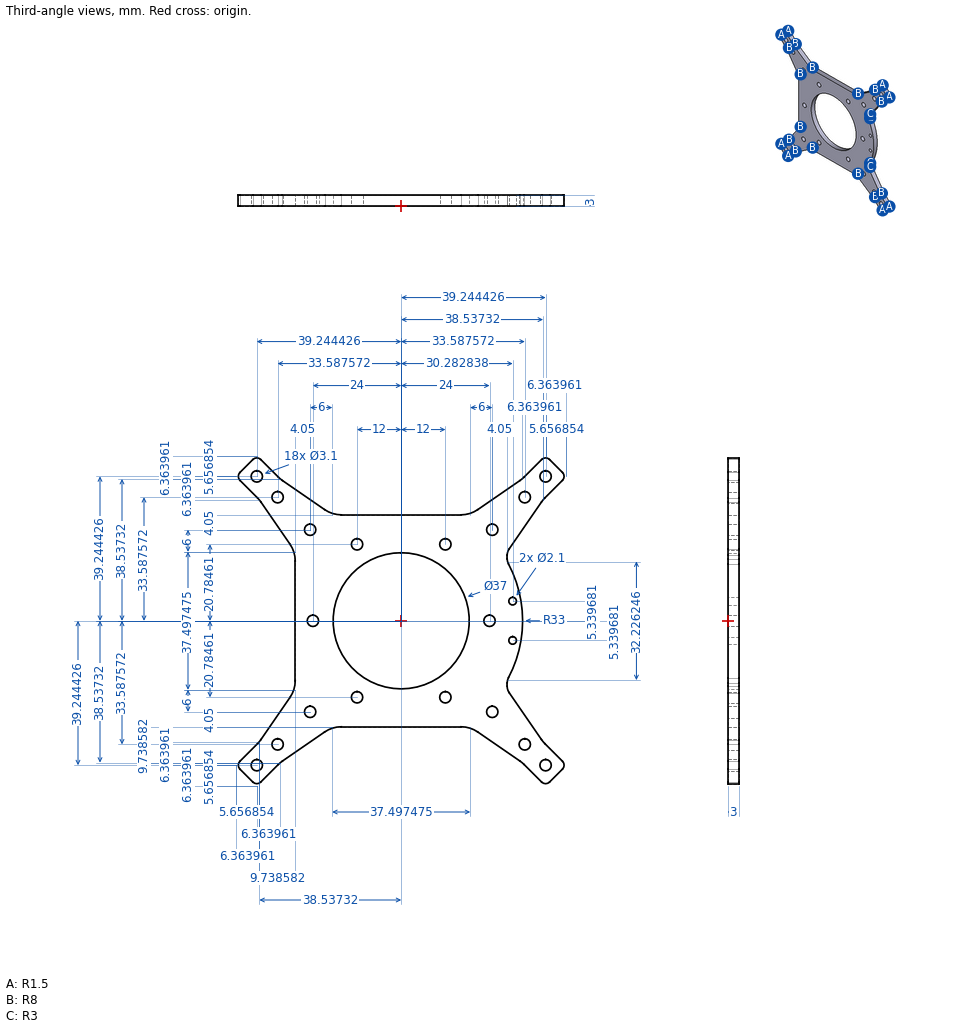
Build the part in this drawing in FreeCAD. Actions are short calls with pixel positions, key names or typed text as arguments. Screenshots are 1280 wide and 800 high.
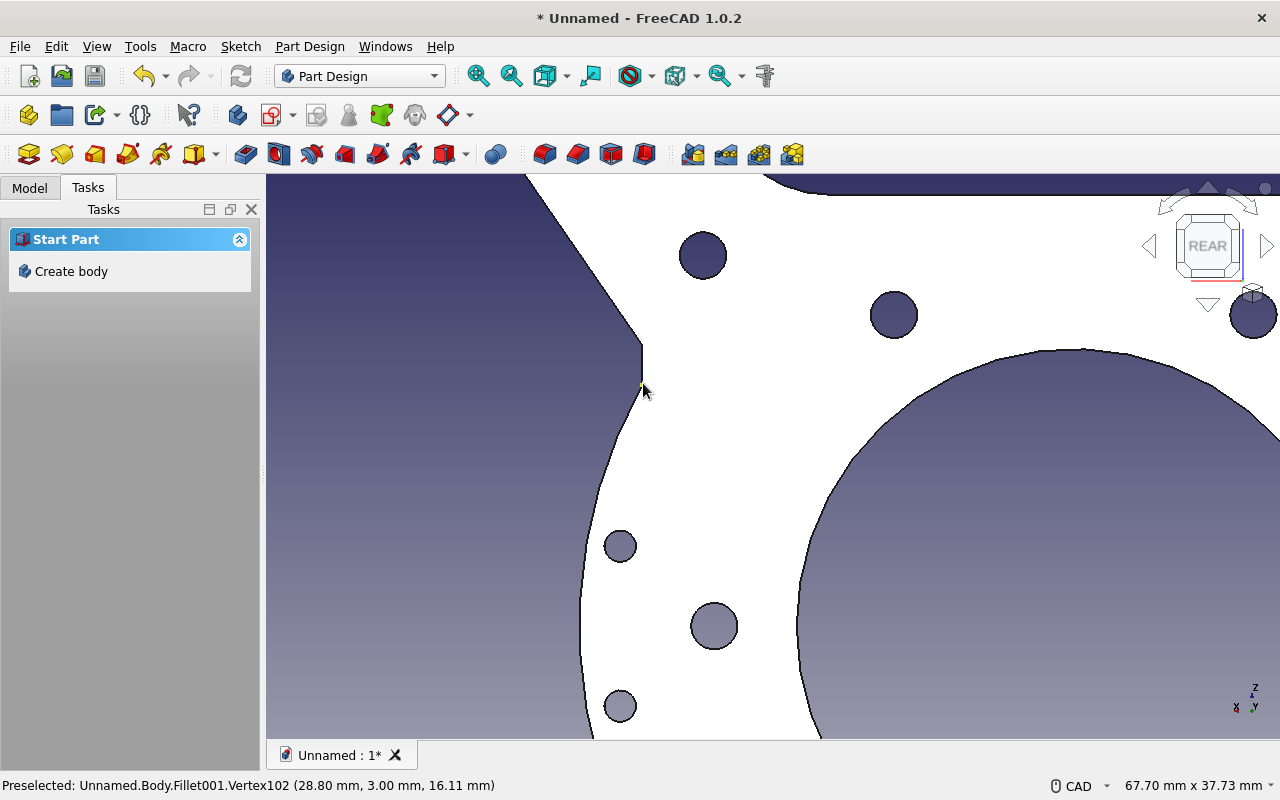
key(v)
key(f)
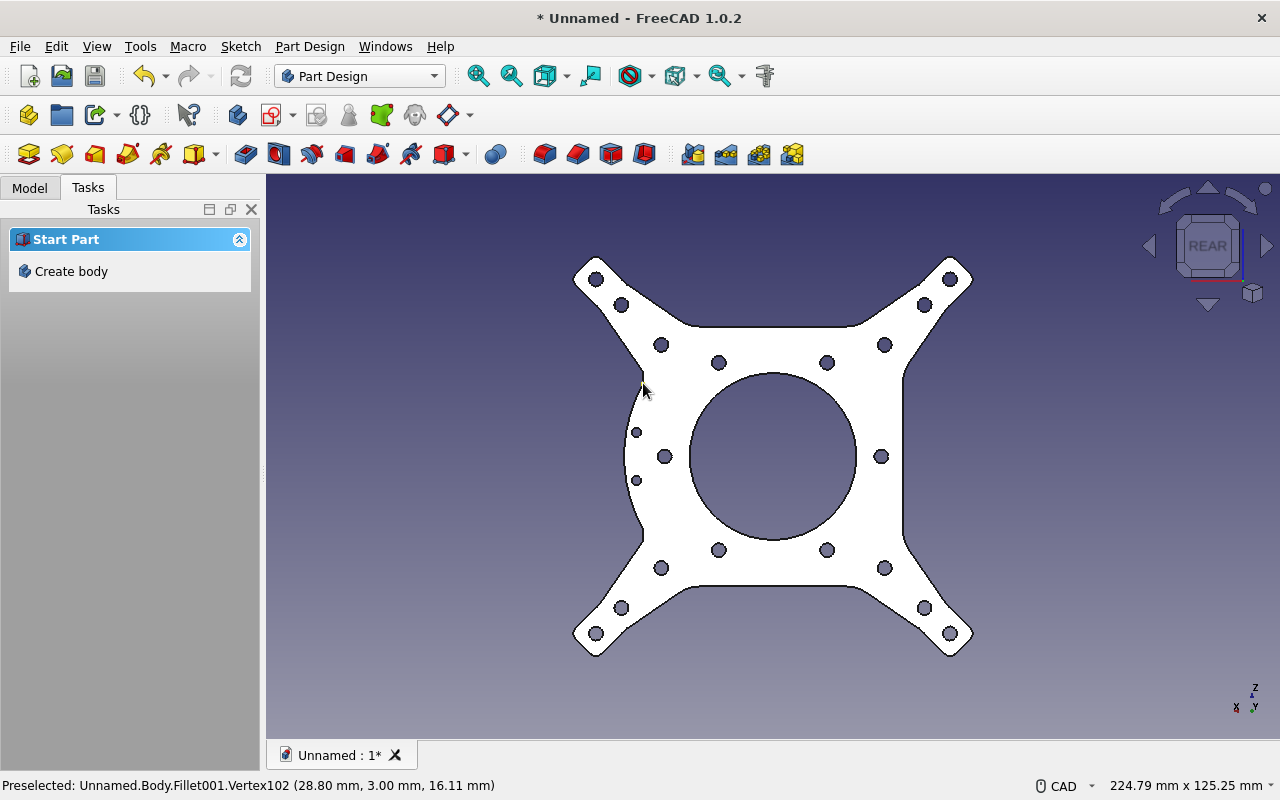
key(6)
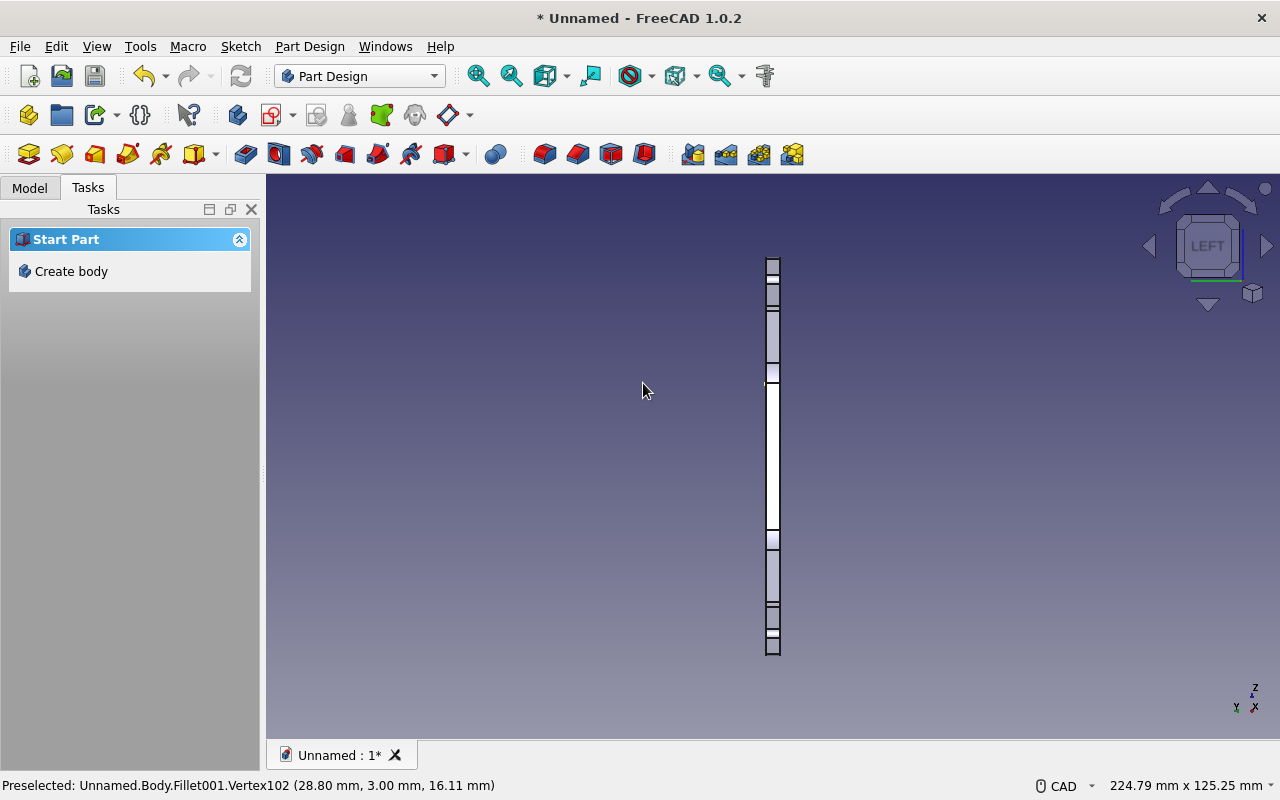
scroll(773, 383, up, 6)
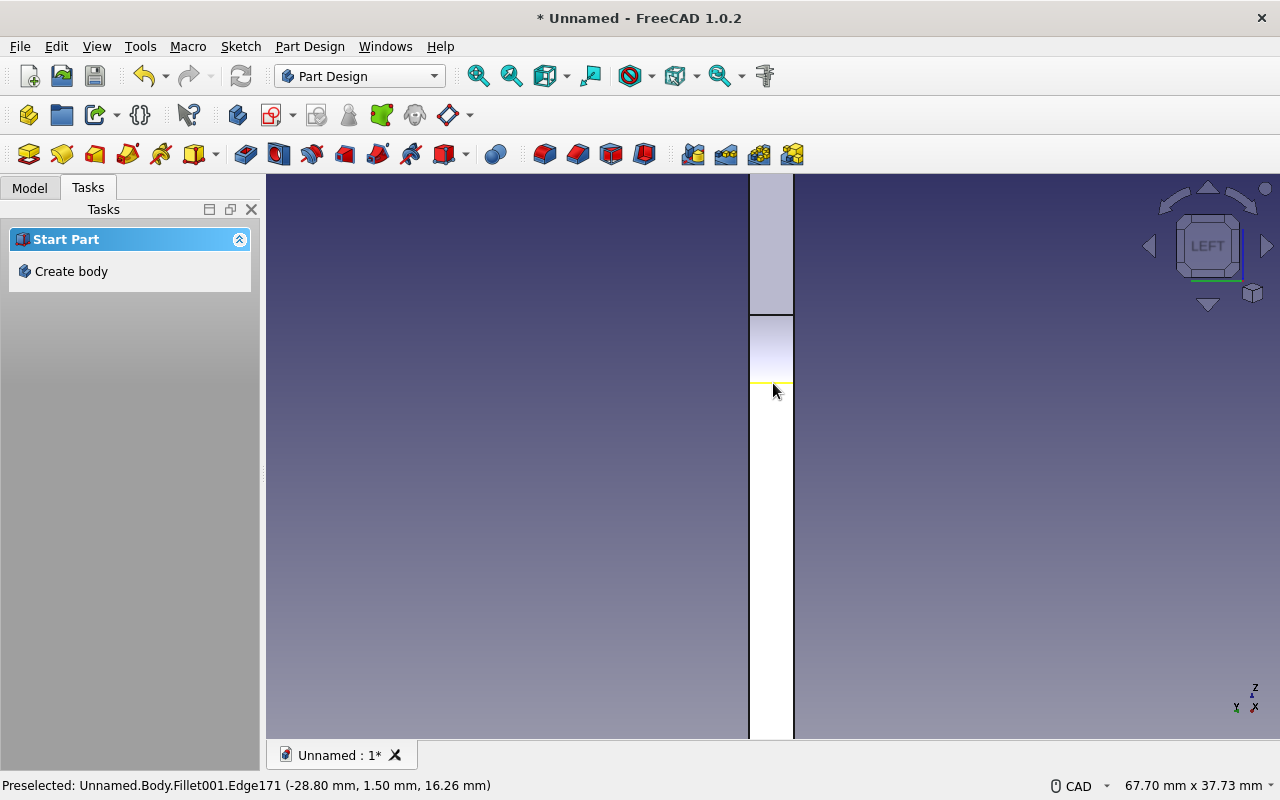
click(479, 76)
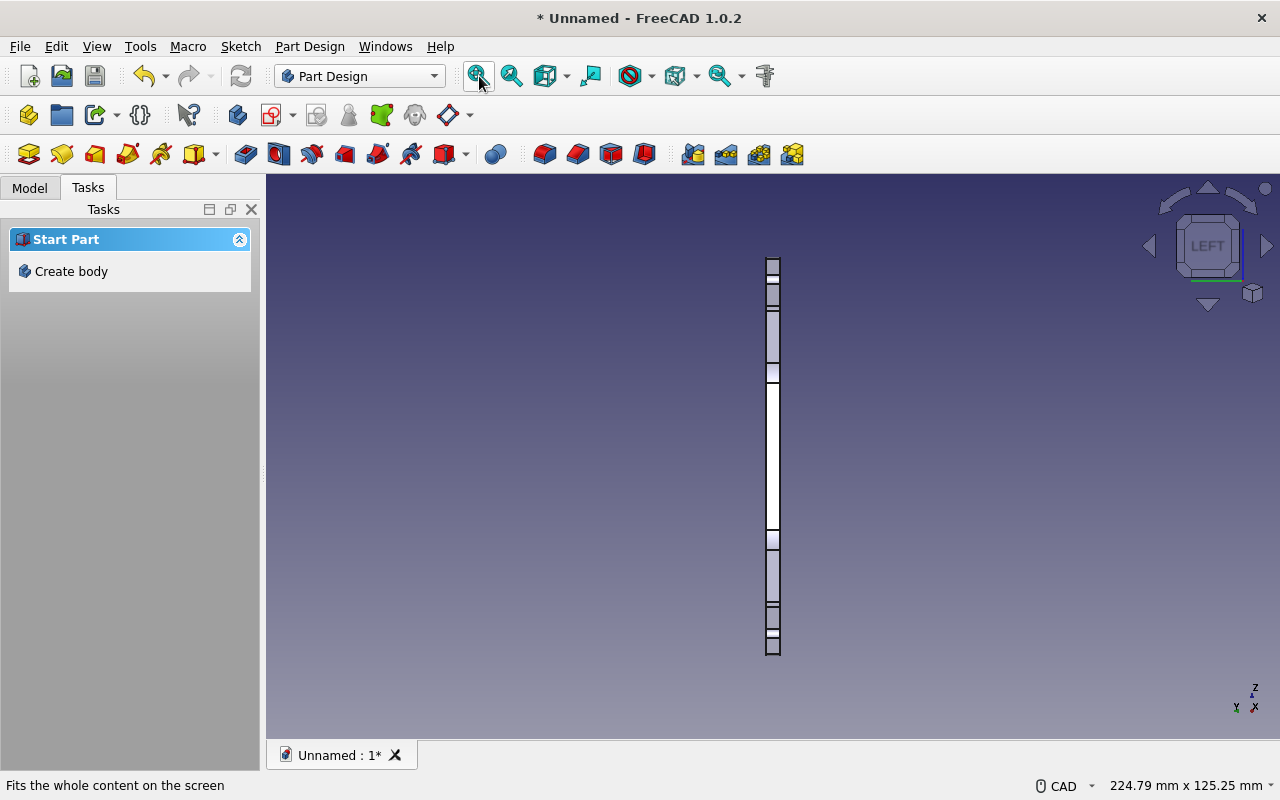
key(v)
key(3)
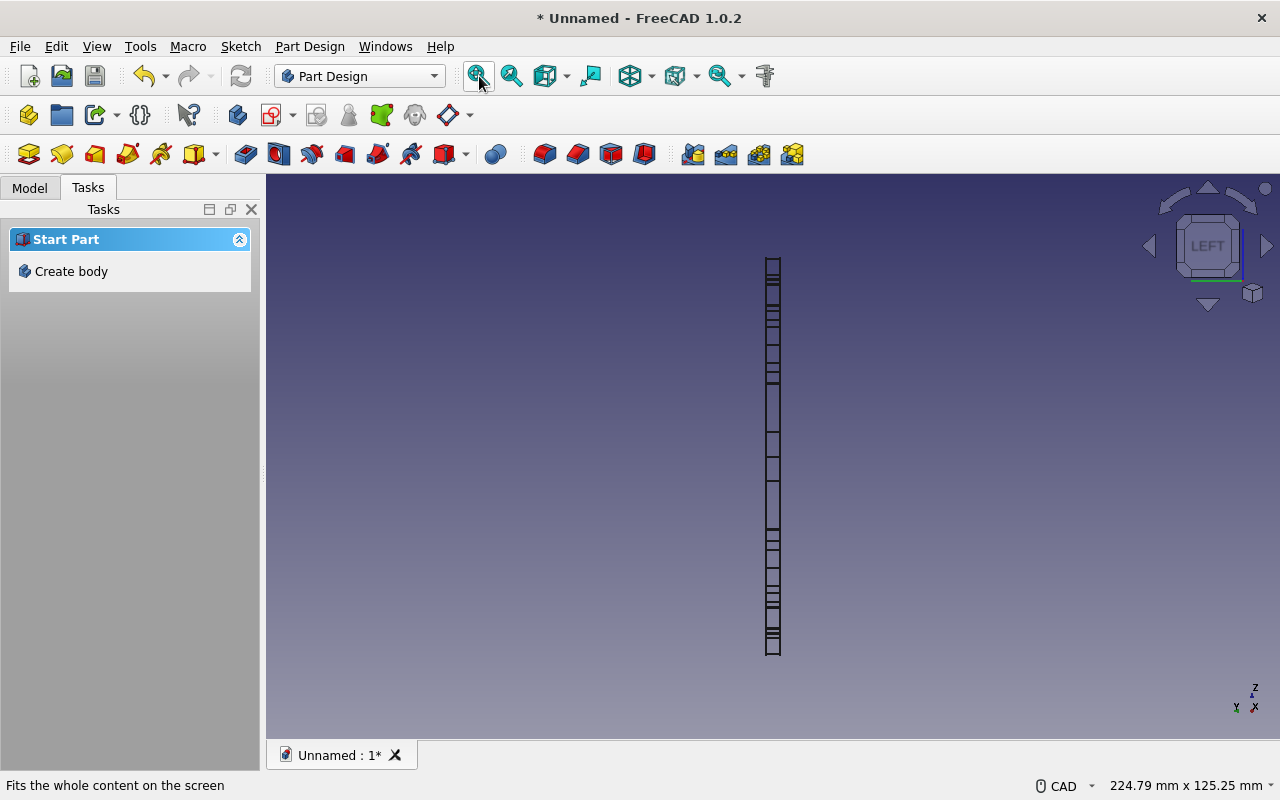
key(0)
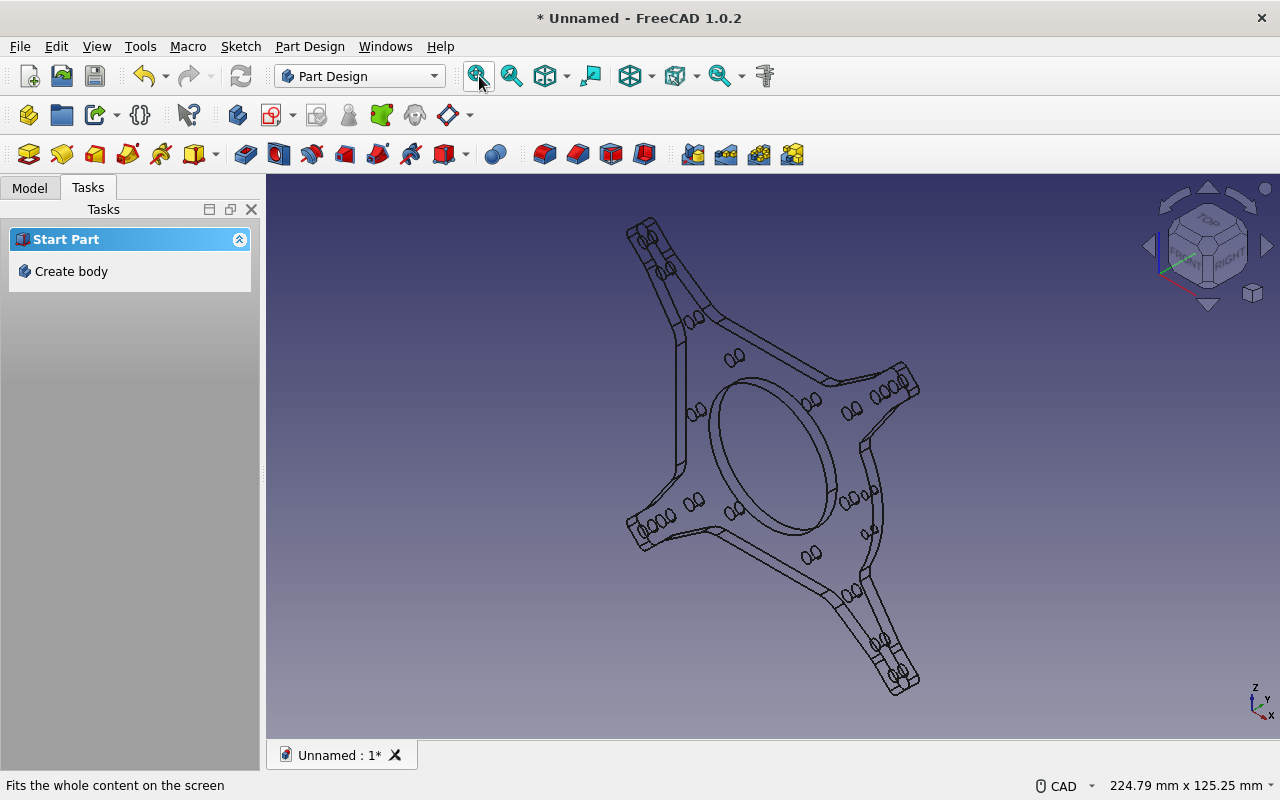
click(867, 448)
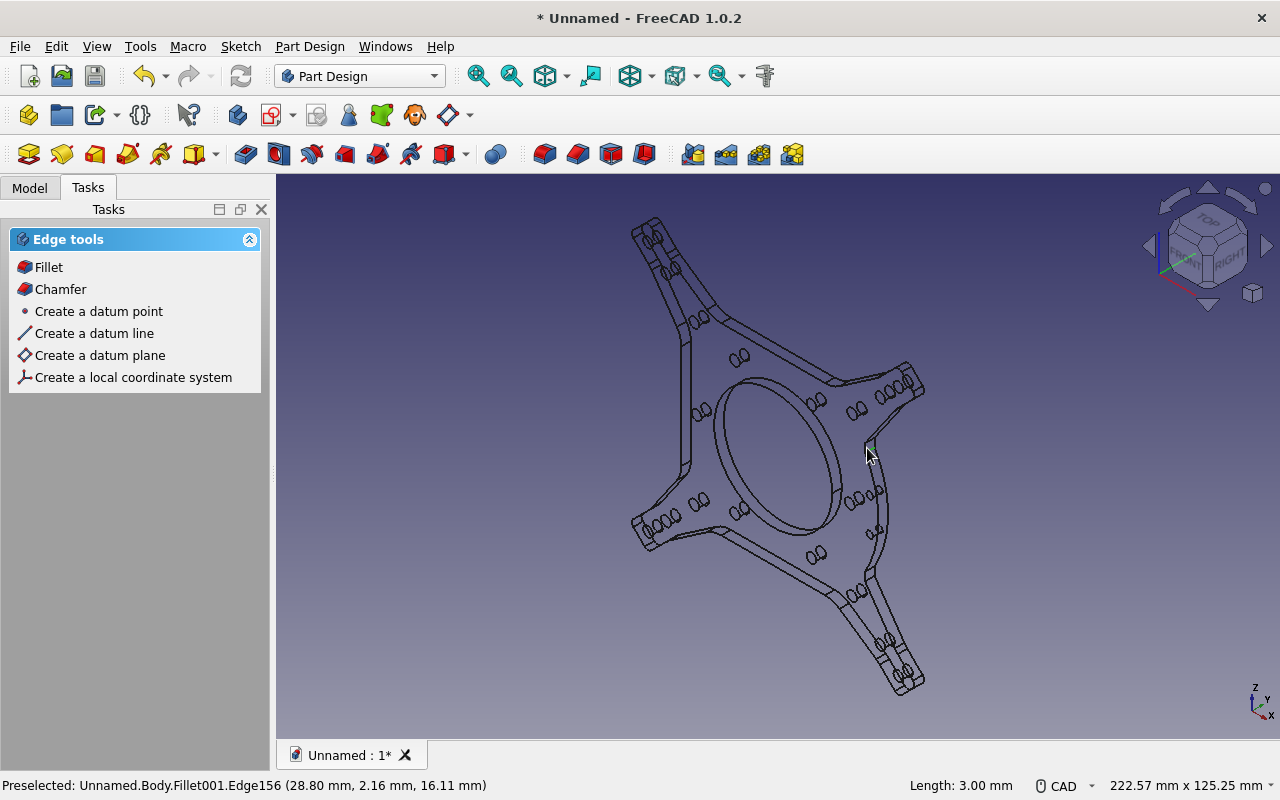
click(872, 576, ctrl)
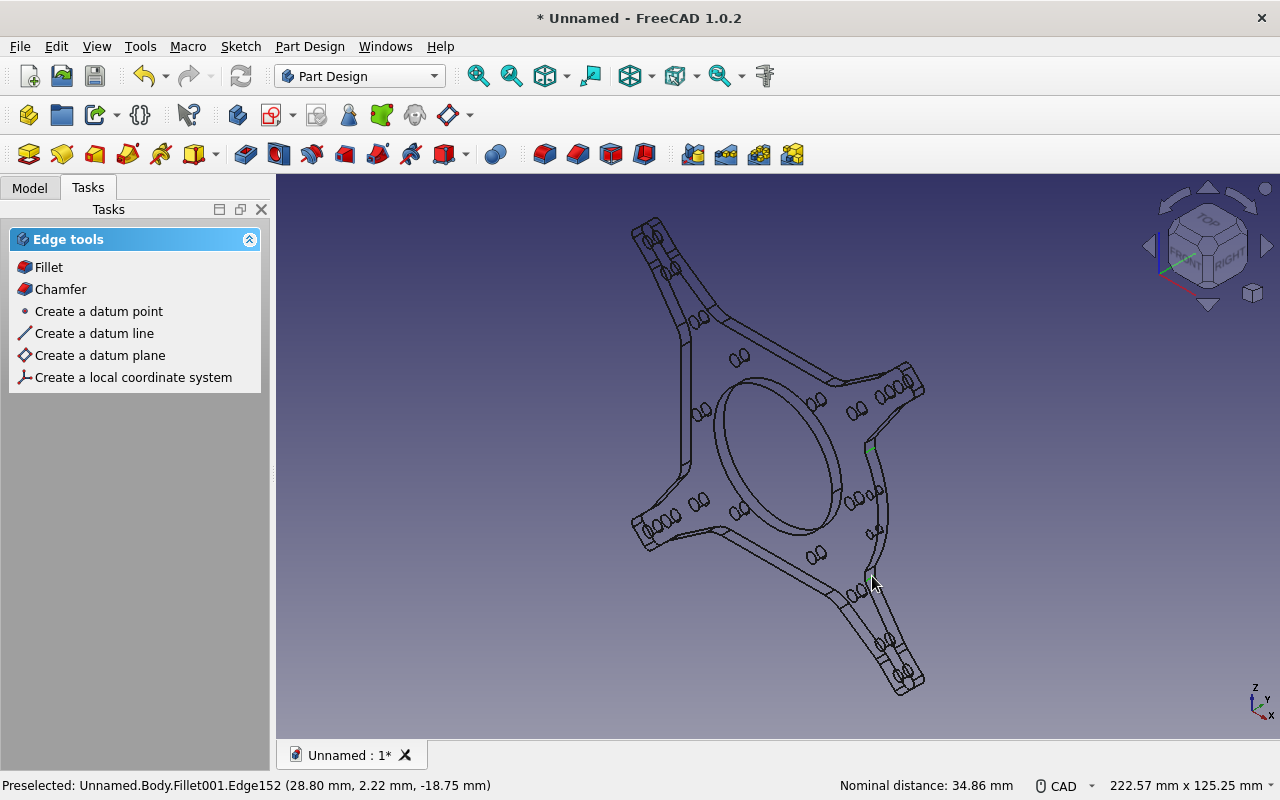
scroll(870, 568, up, 6)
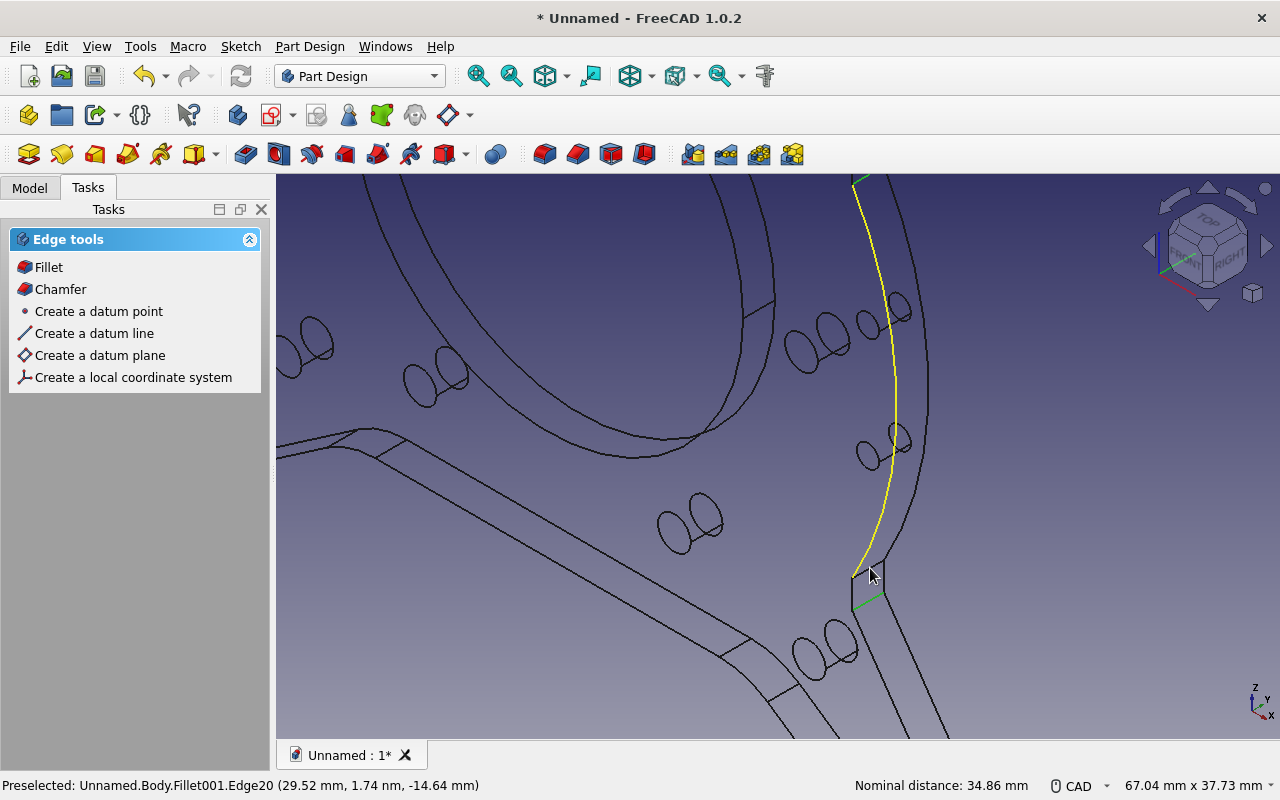
click(868, 568, ctrl)